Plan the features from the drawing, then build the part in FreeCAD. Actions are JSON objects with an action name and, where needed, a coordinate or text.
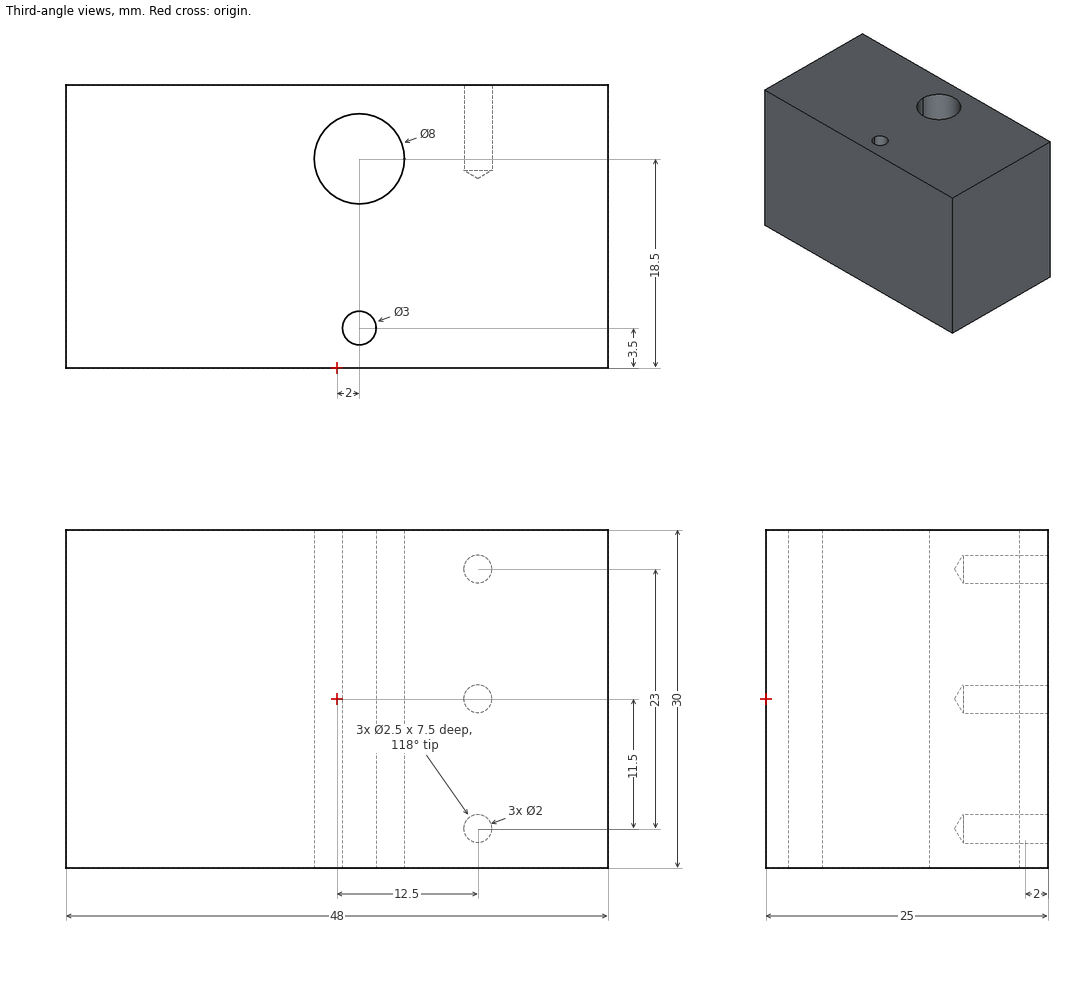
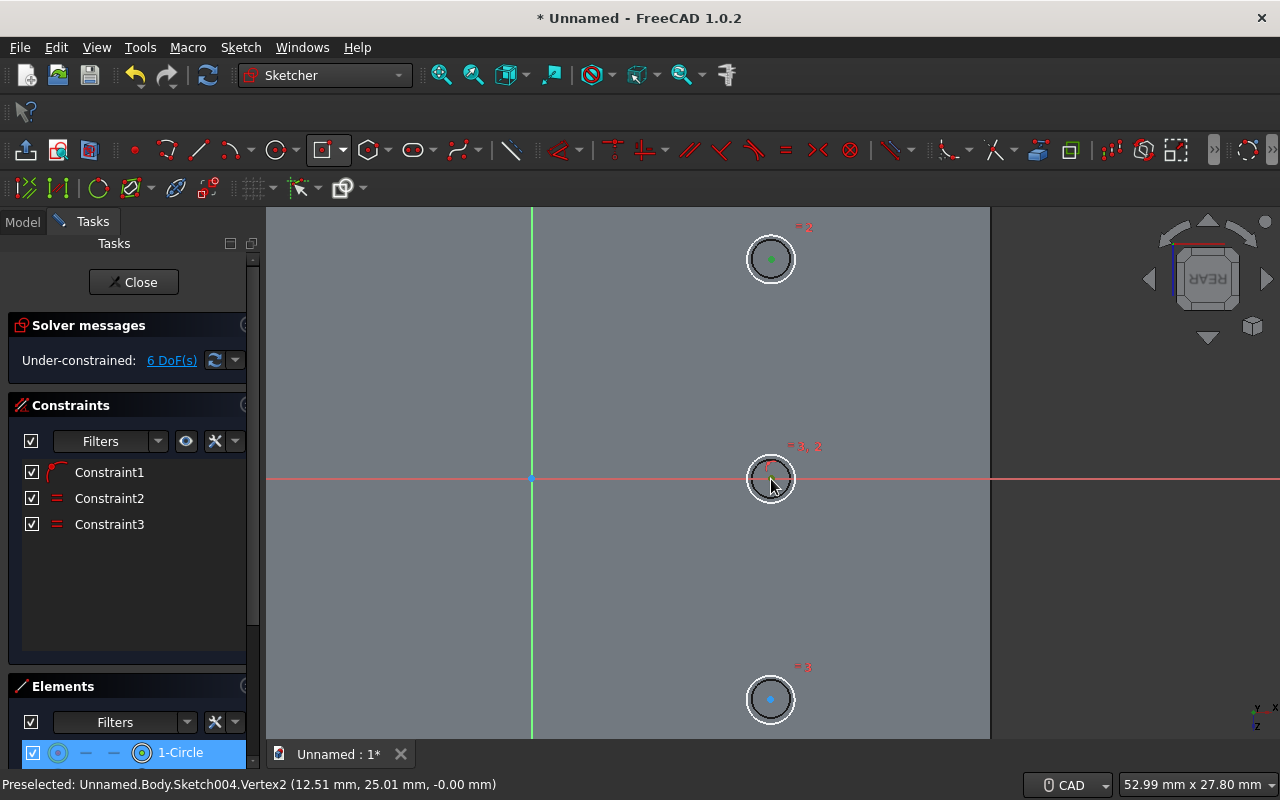
{"action": "left_click", "coordinate": [668, 150]}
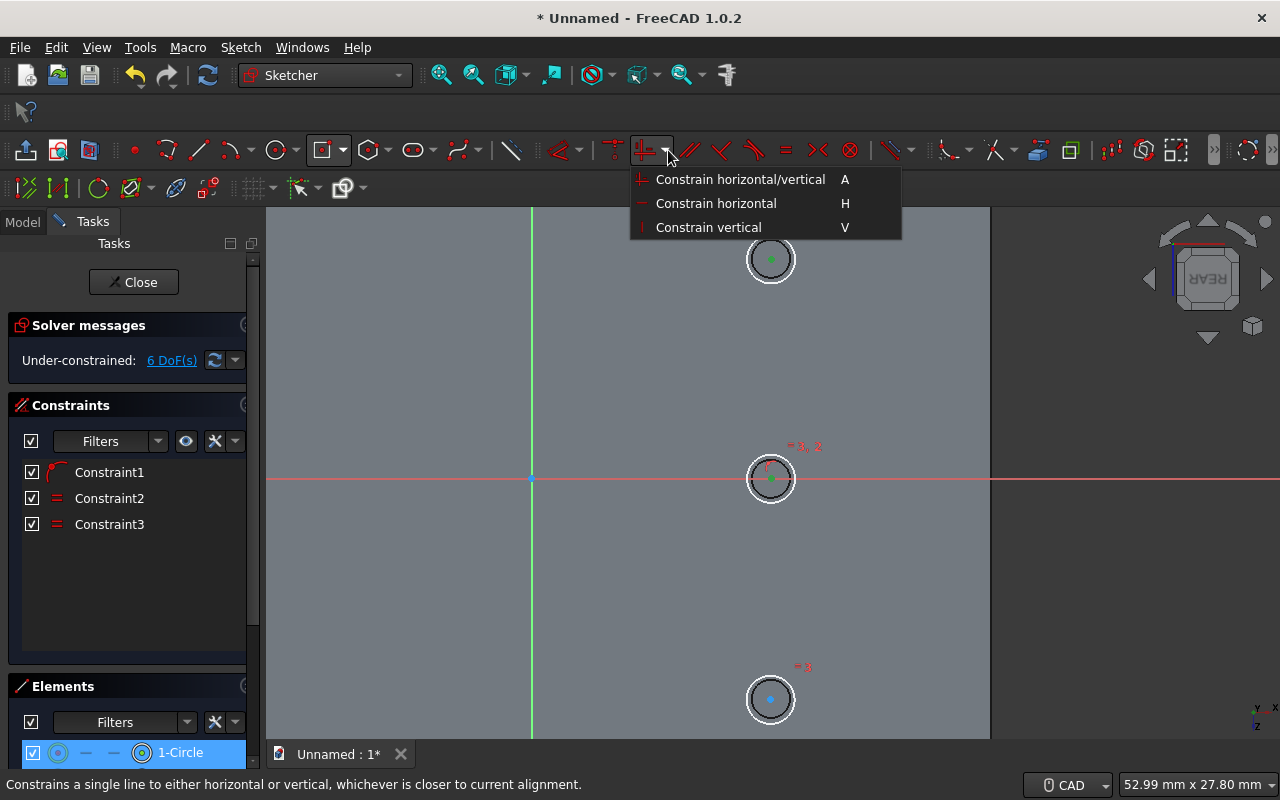
{"action": "left_click", "coordinate": [766, 227]}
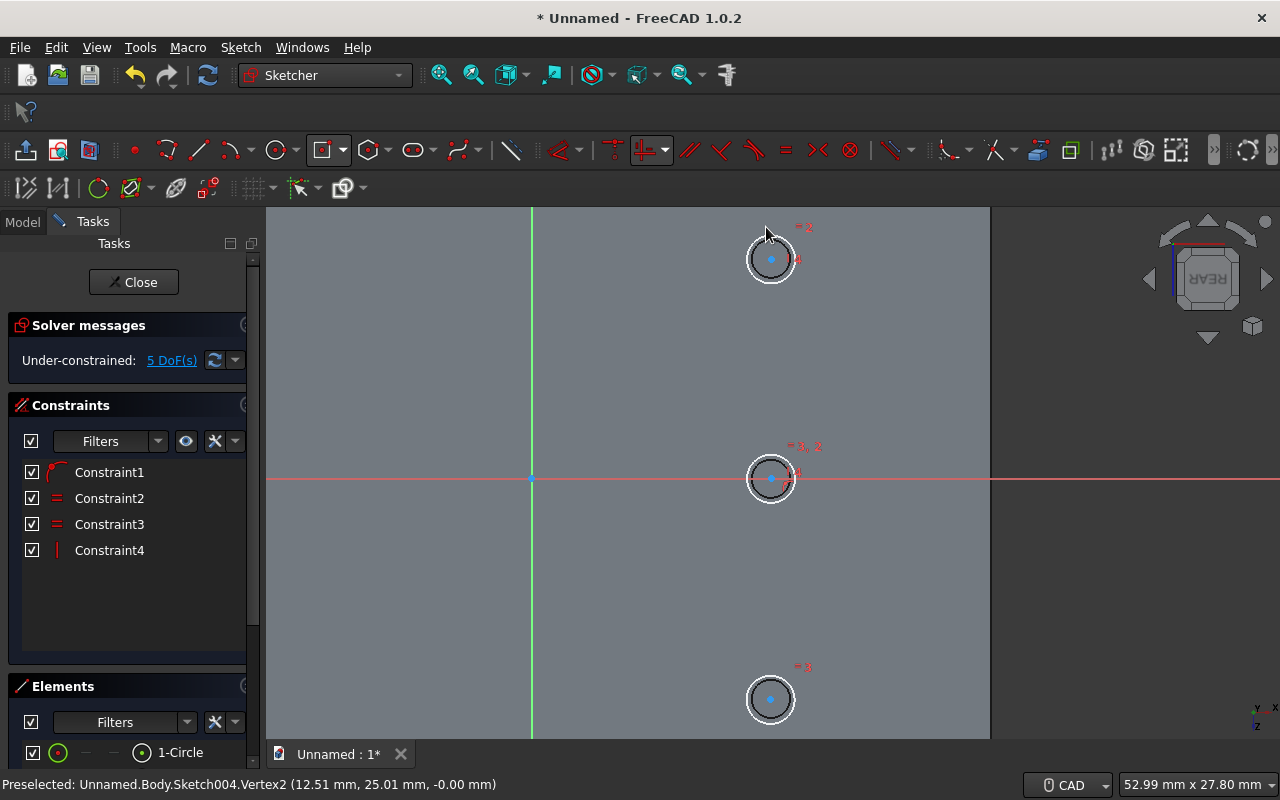
{"action": "left_click", "coordinate": [771, 479]}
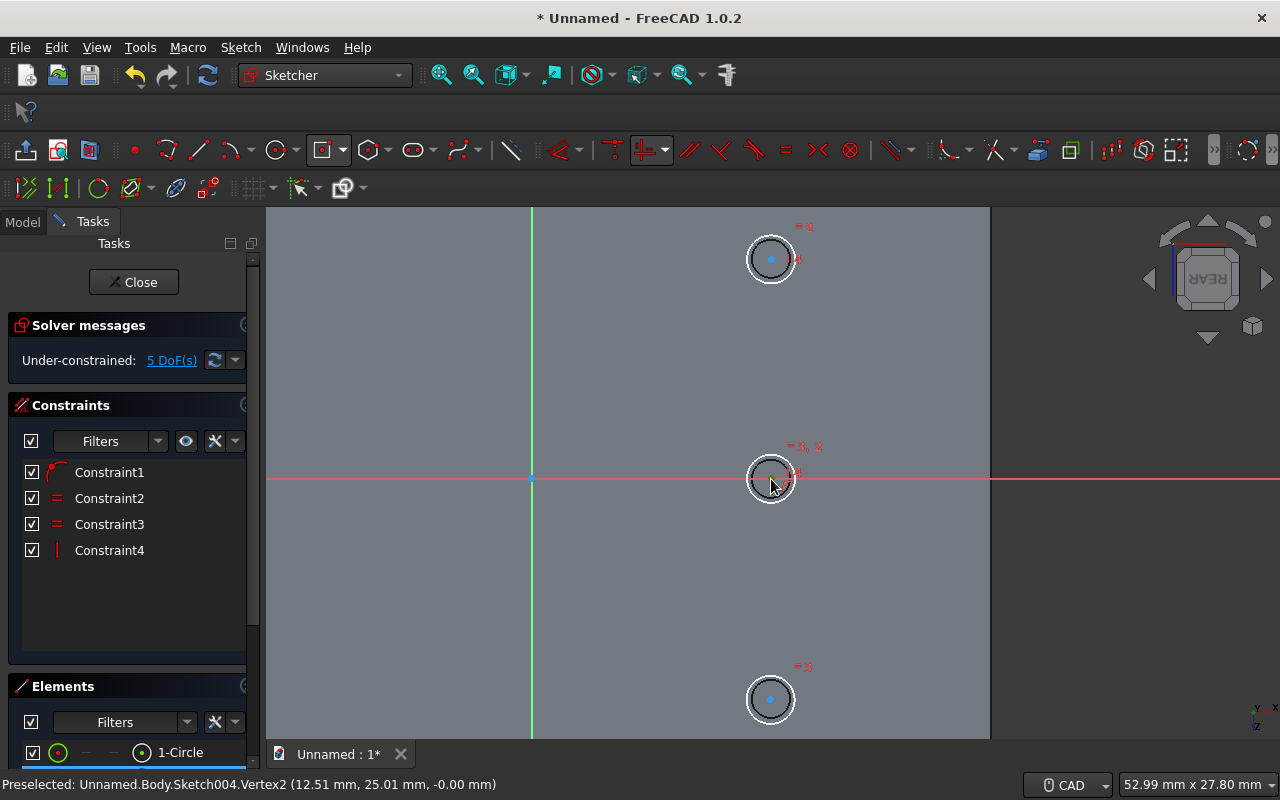
{"action": "left_click", "coordinate": [771, 700]}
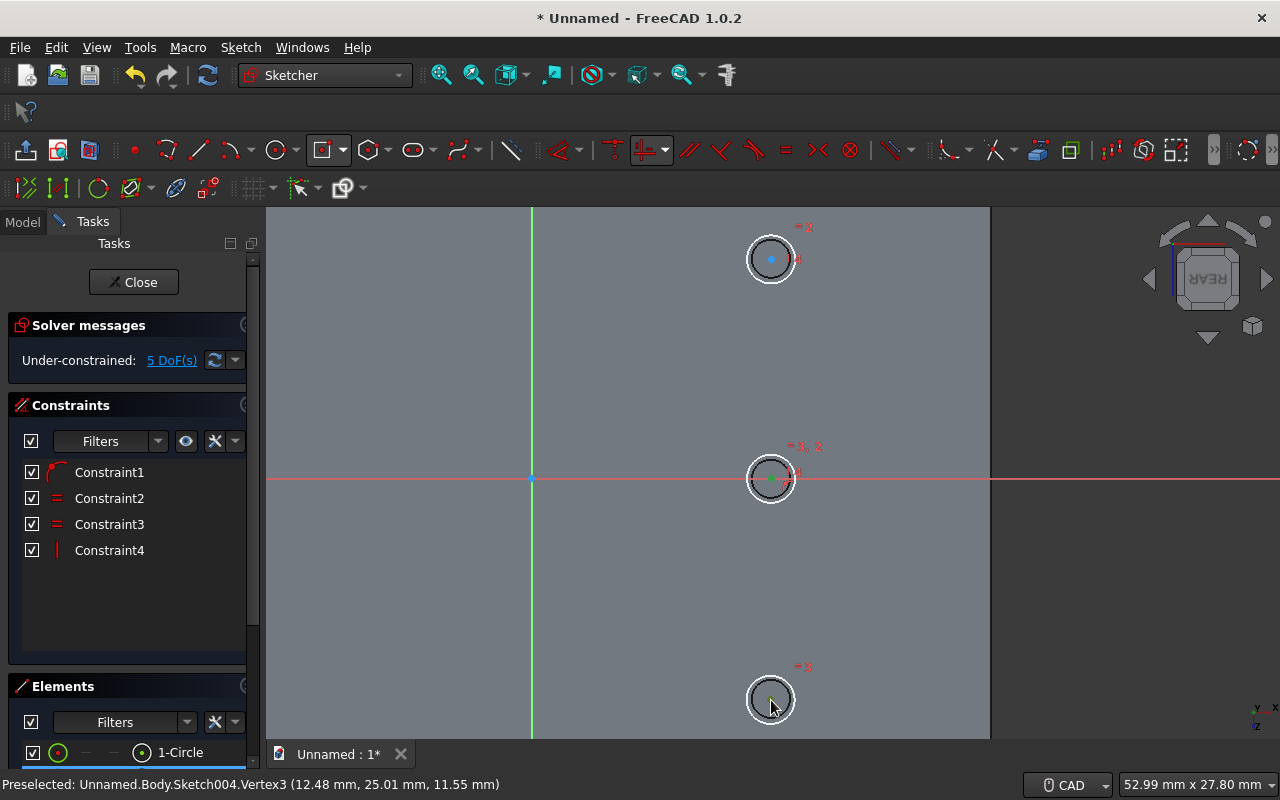
{"action": "key", "text": "v"}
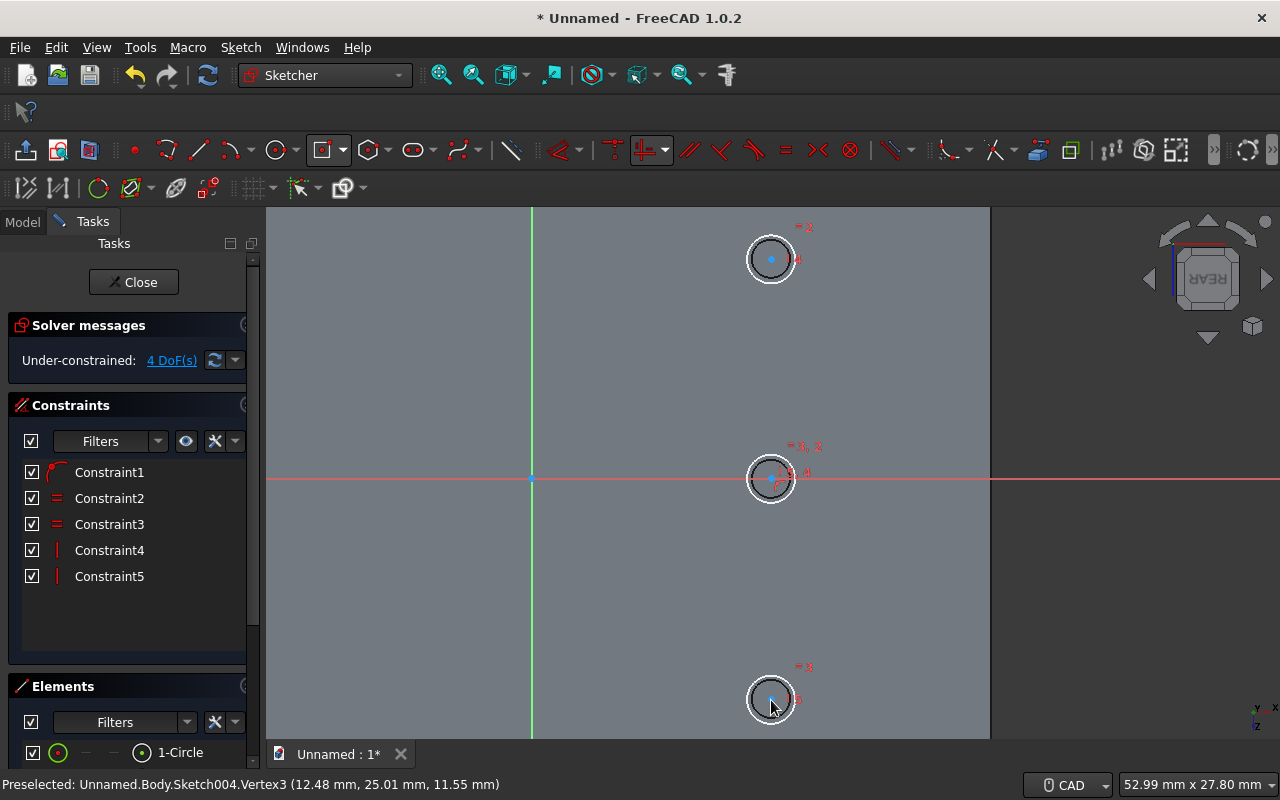
{"action": "key", "text": "d"}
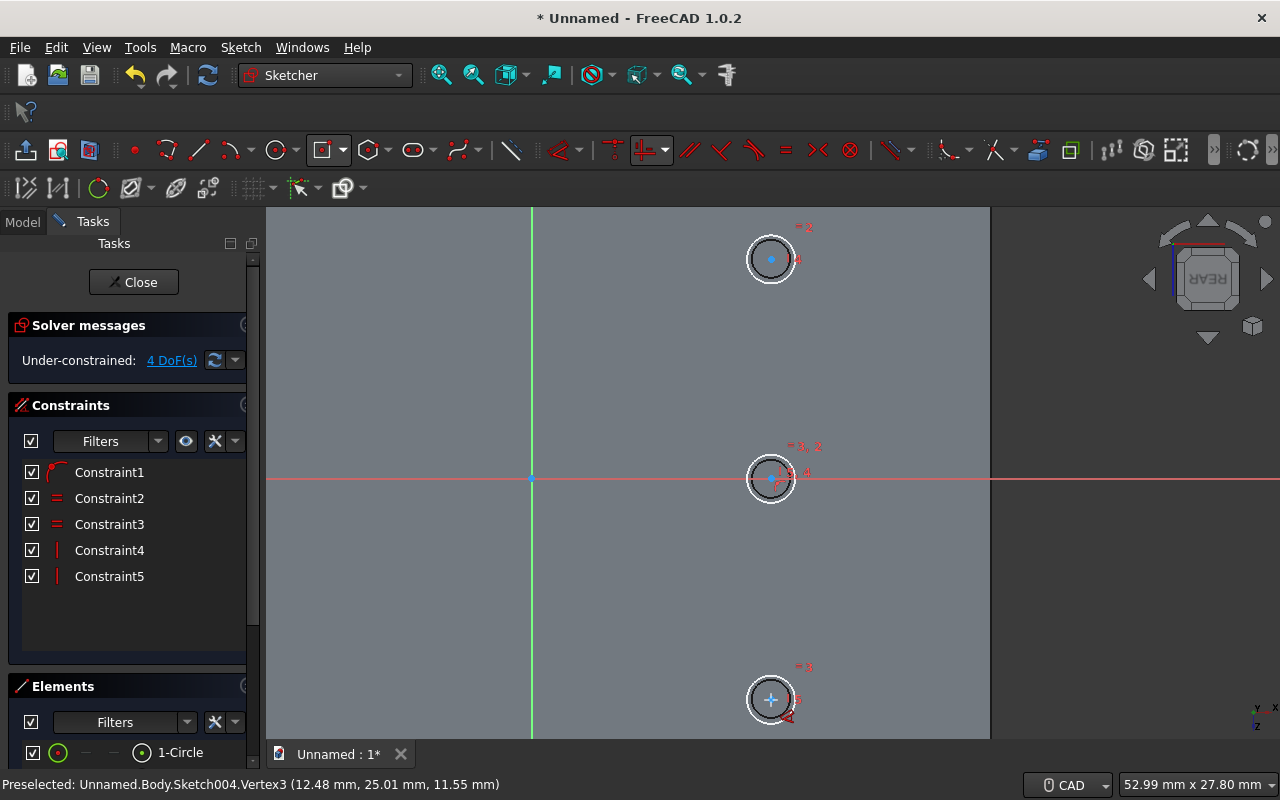
{"action": "left_click", "coordinate": [788, 242]}
{"action": "left_click", "coordinate": [825, 243]}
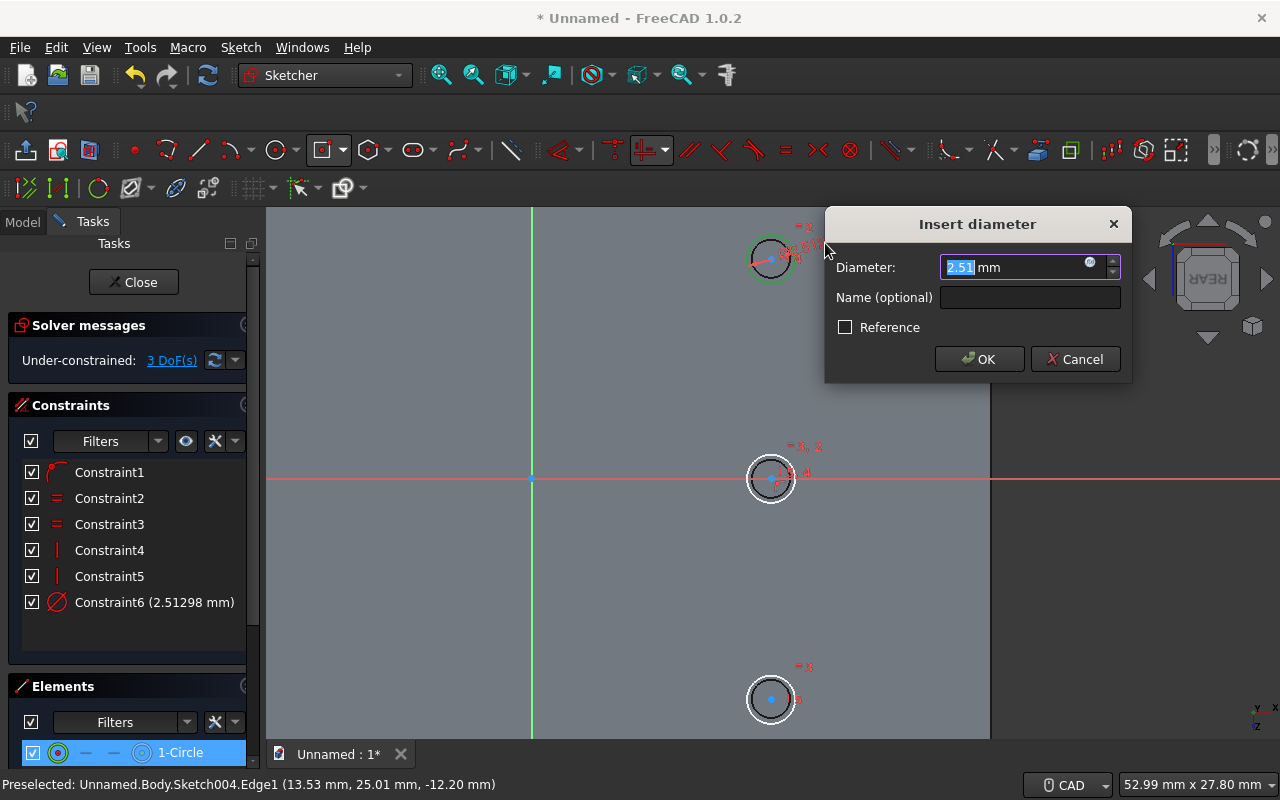
{"action": "type", "text": "2.5"}
{"action": "key", "text": "Return"}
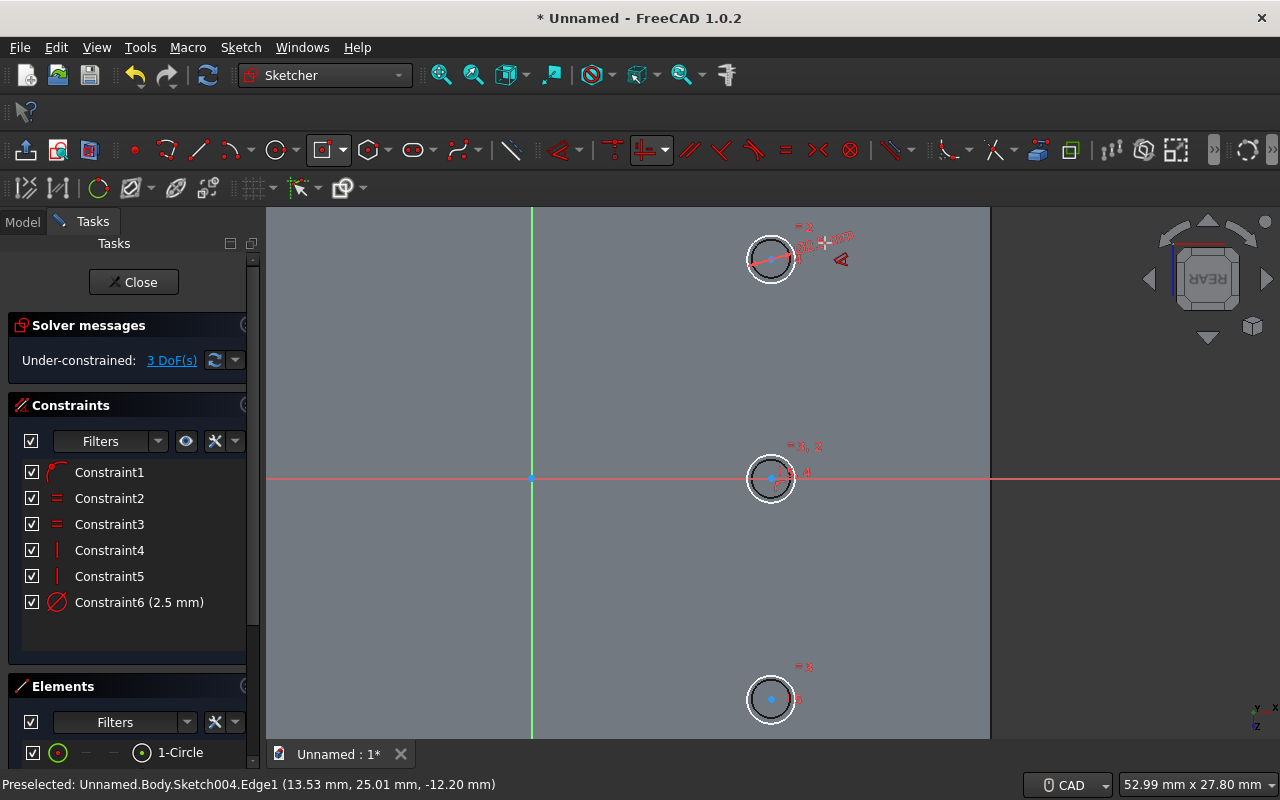
{"action": "left_click", "coordinate": [771, 259]}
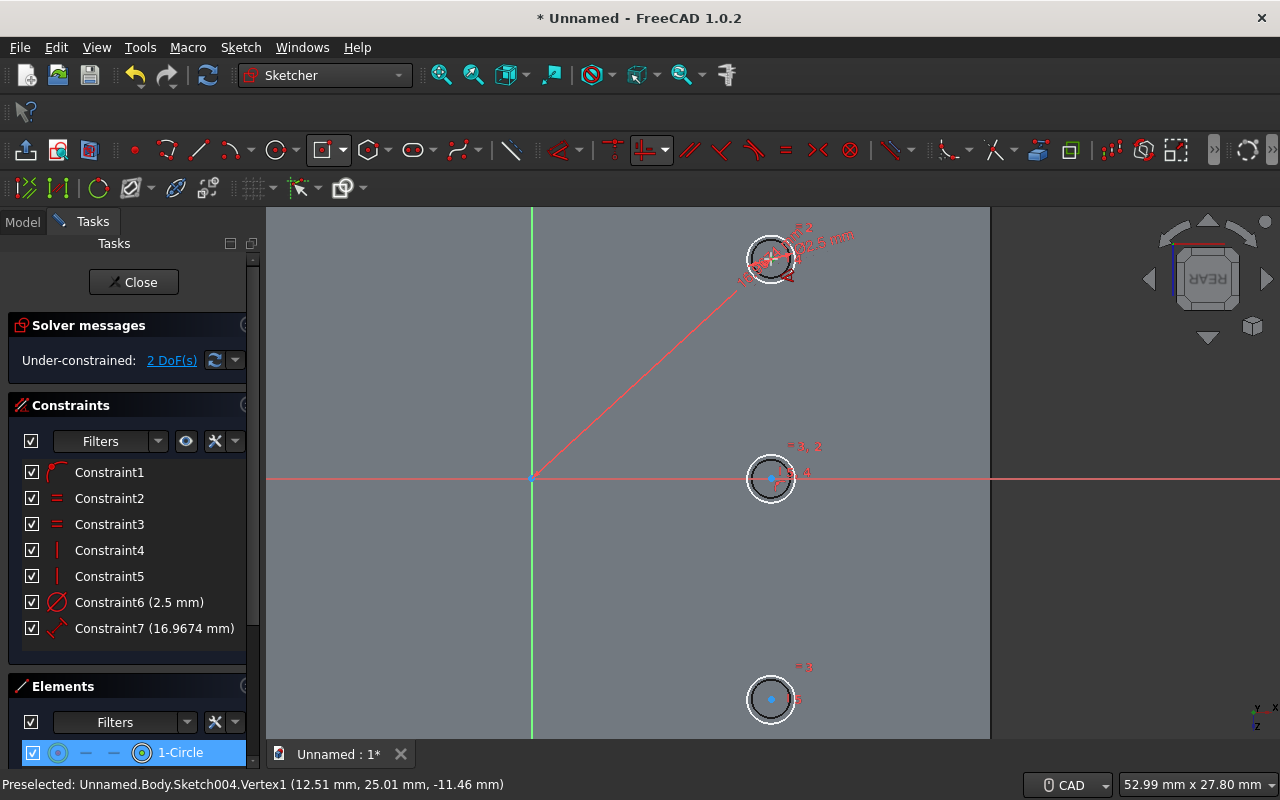
{"action": "left_click", "coordinate": [771, 700]}
{"action": "left_click", "coordinate": [805, 378]}